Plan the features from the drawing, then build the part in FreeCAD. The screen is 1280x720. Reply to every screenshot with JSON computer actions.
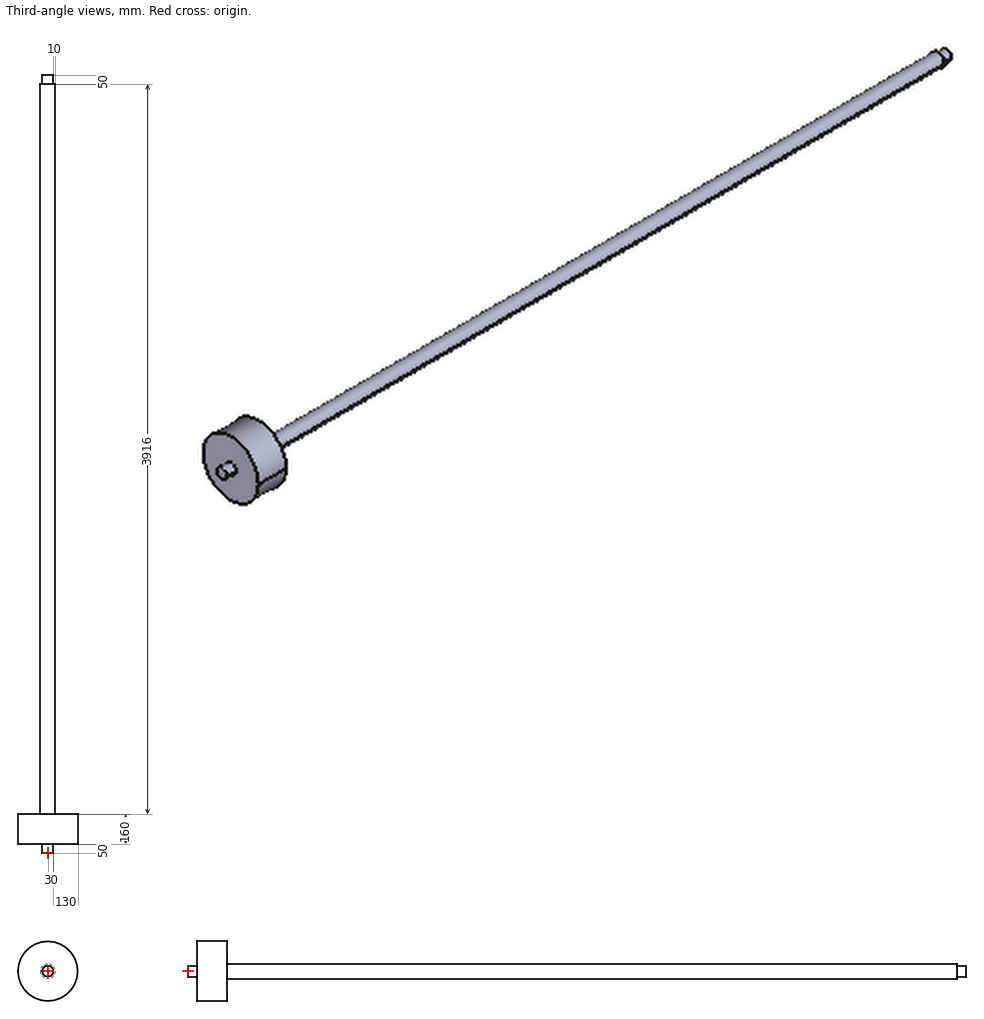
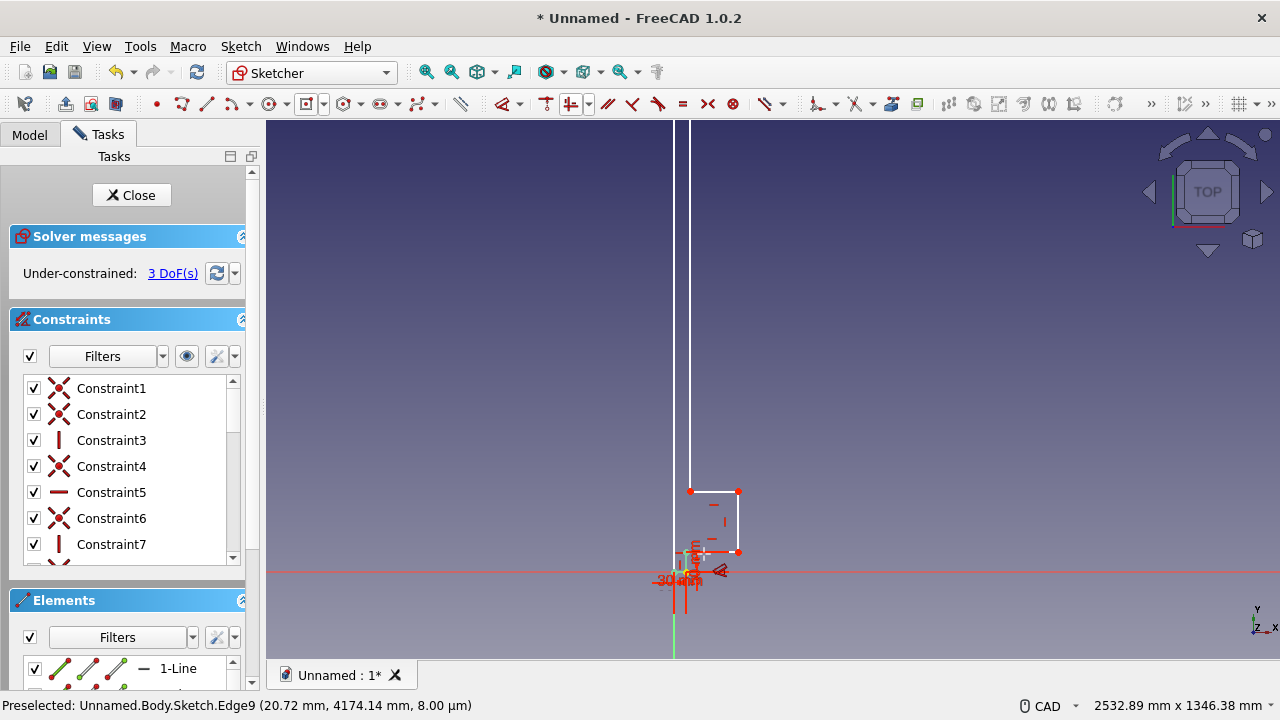
{"action": "left_click", "coordinate": [702, 552]}
{"action": "left_click", "coordinate": [712, 518]}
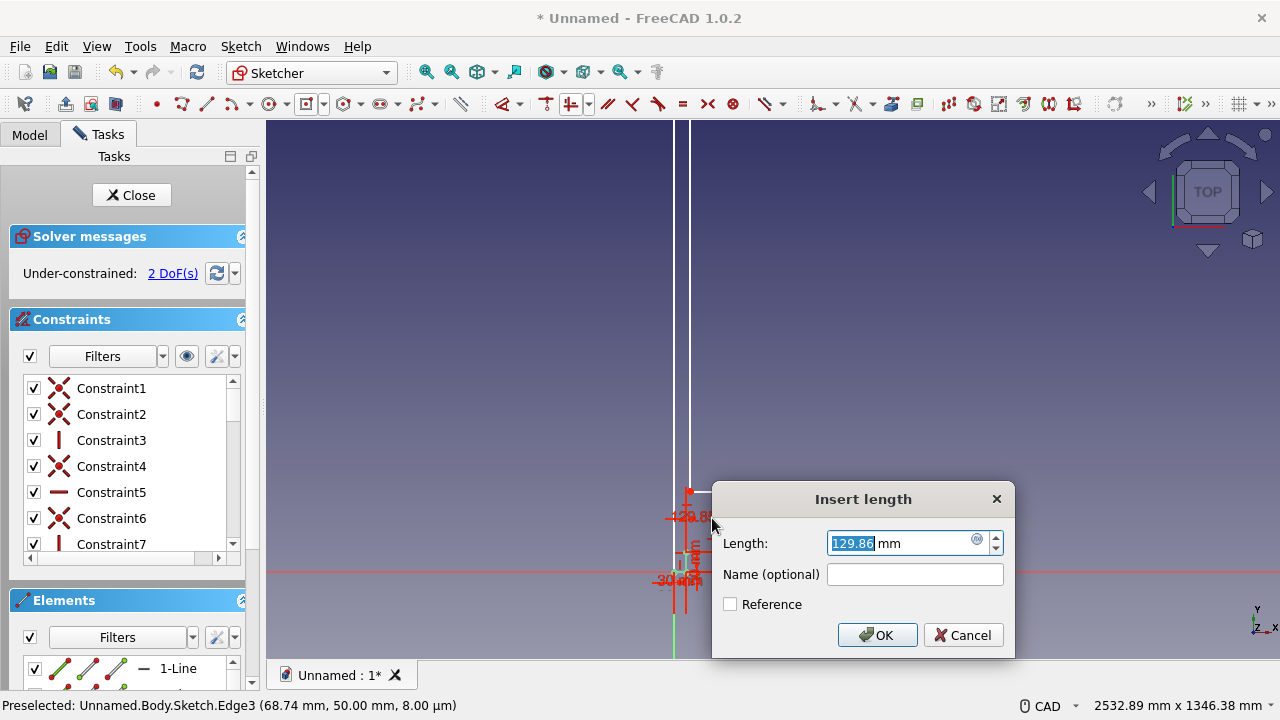
{"action": "type", "text": "130"}
{"action": "key", "text": "Return"}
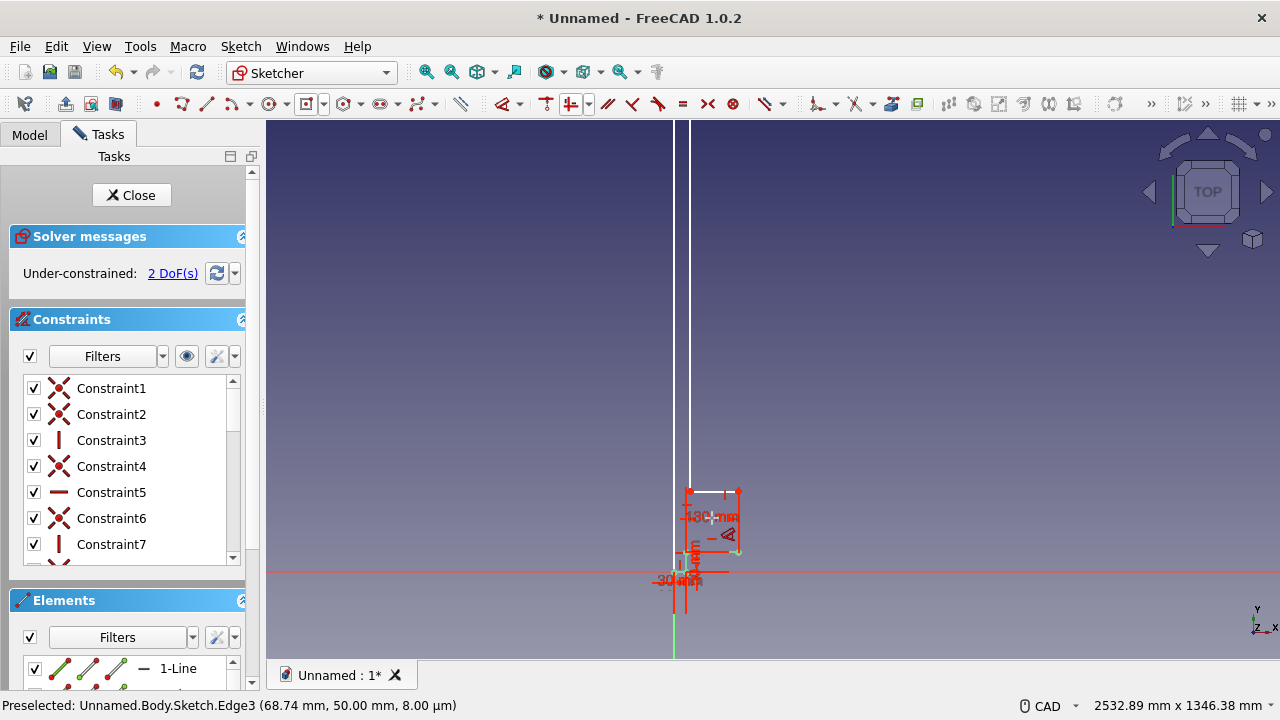
{"action": "left_click", "coordinate": [739, 534]}
{"action": "left_click", "coordinate": [773, 543]}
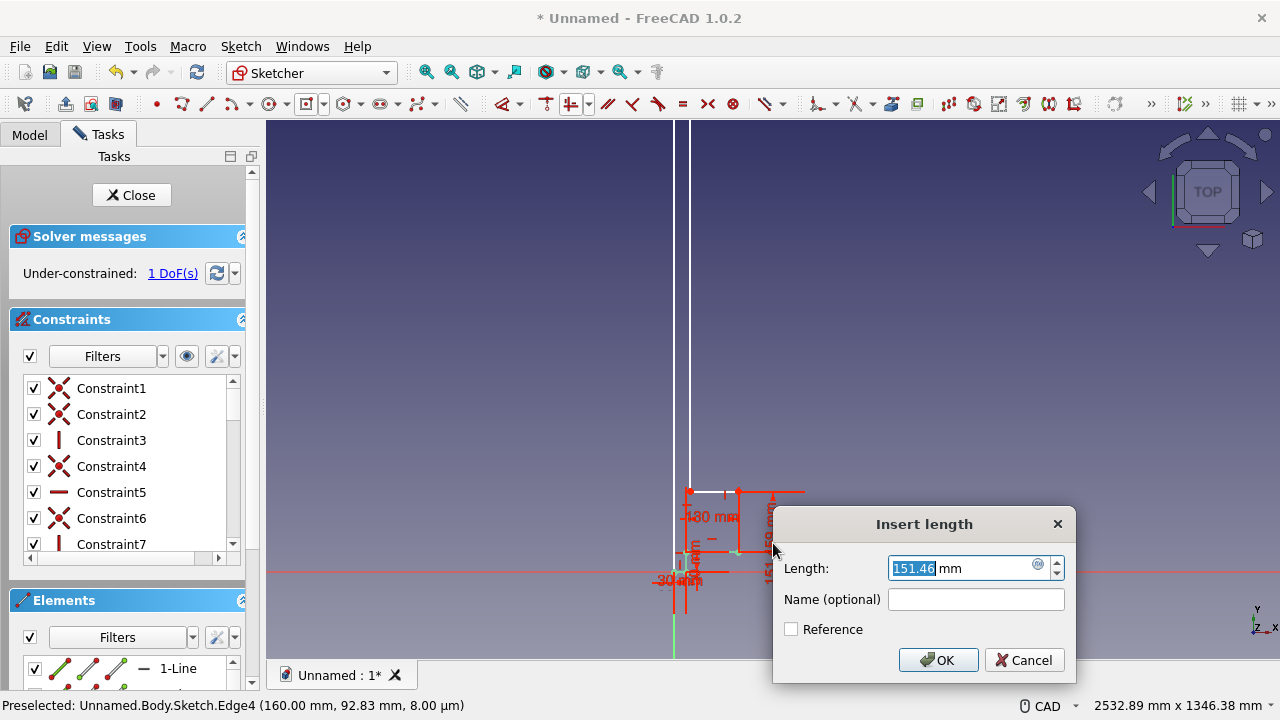
{"action": "type", "text": "160"}
{"action": "key", "text": "Return"}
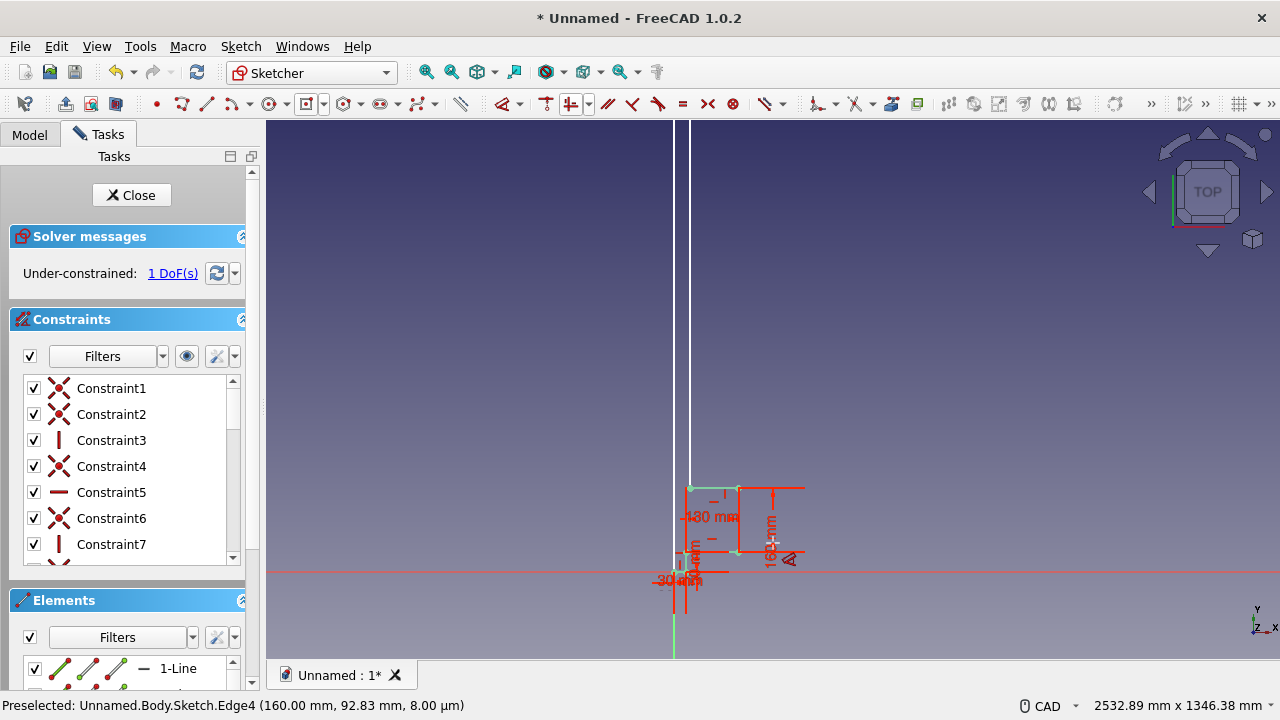
{"action": "left_click", "coordinate": [690, 175]}
{"action": "left_click", "coordinate": [656, 318]}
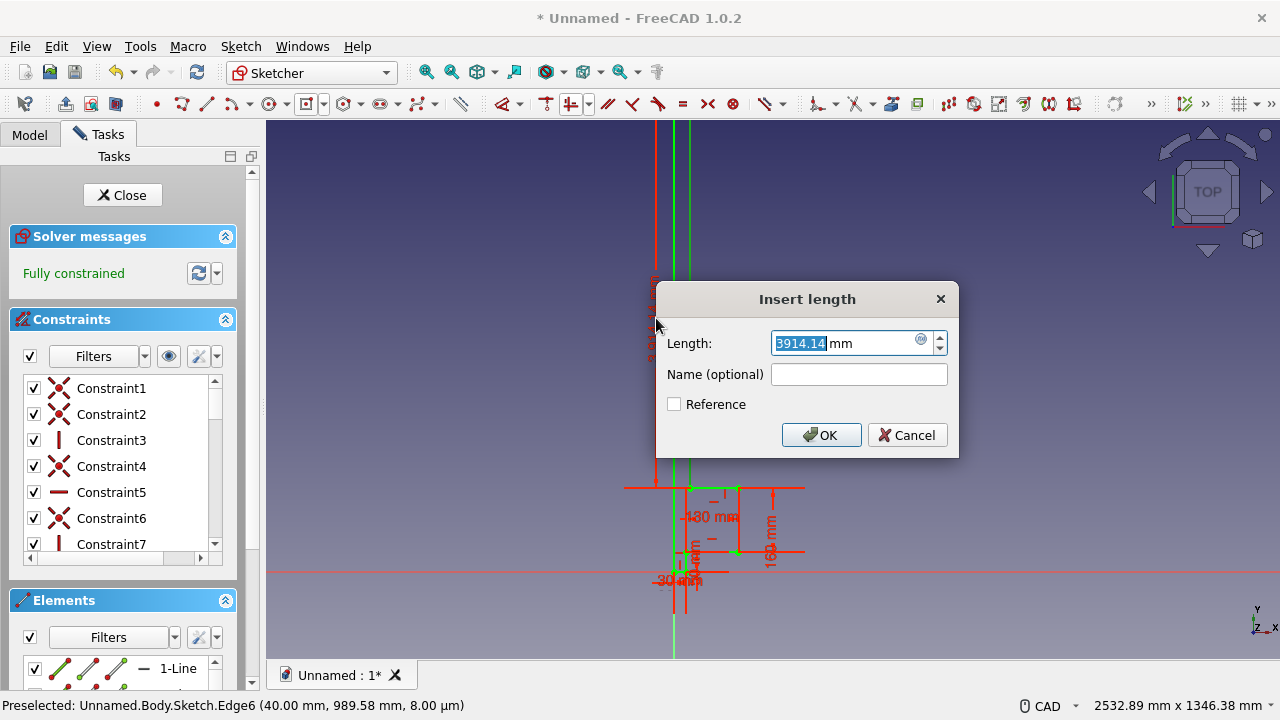
{"action": "type", "text": "3916"}
{"action": "key", "text": "Return"}
{"action": "key", "text": "Escape"}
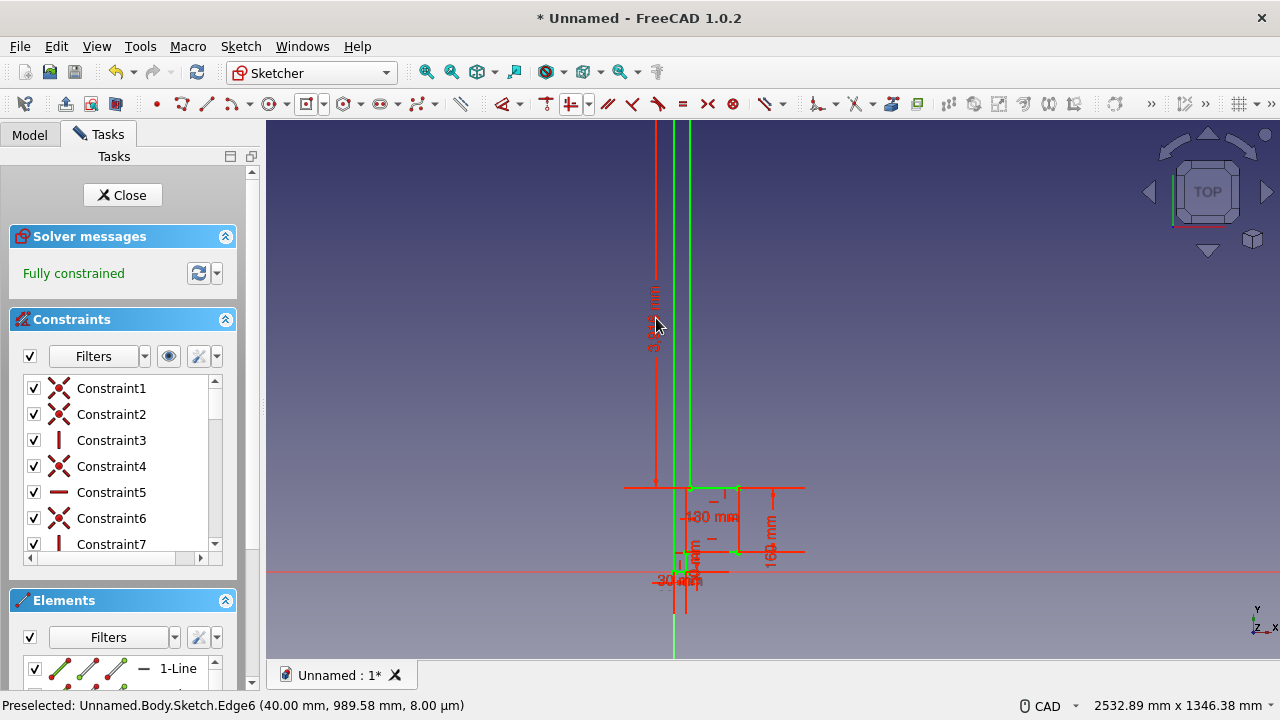
{"action": "left_click", "coordinate": [123, 195]}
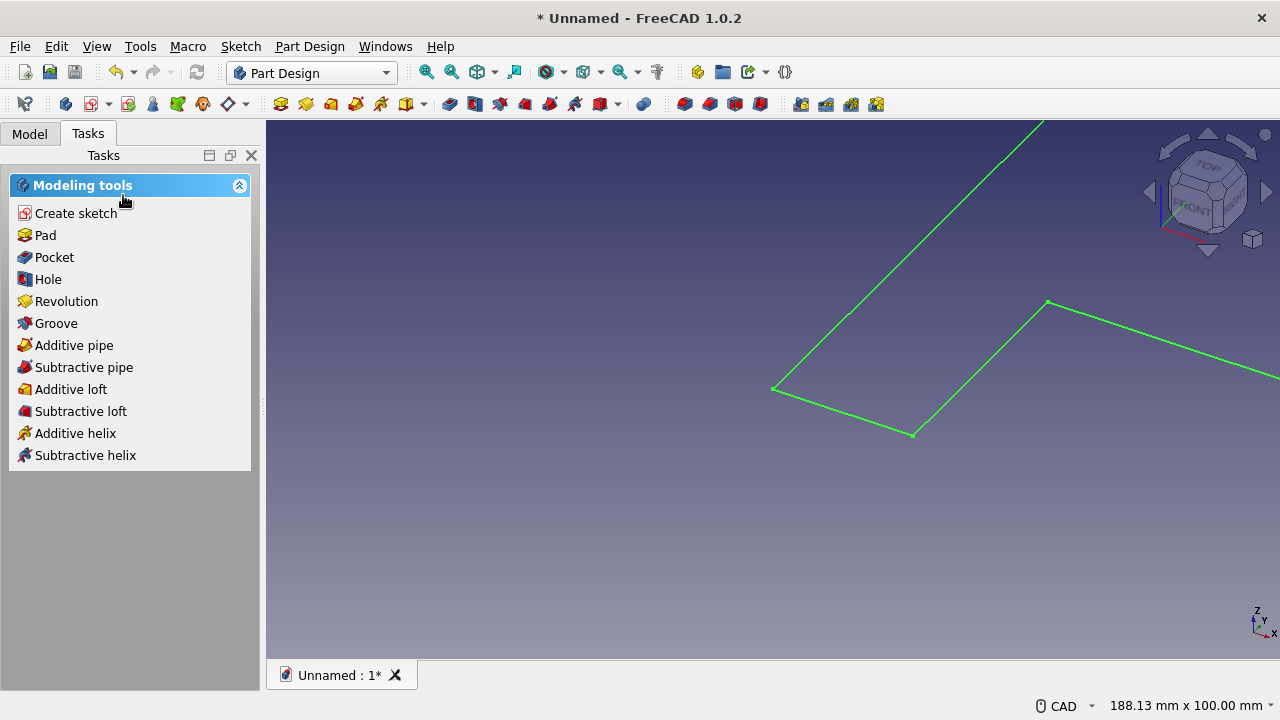
{"action": "left_click", "coordinate": [306, 104]}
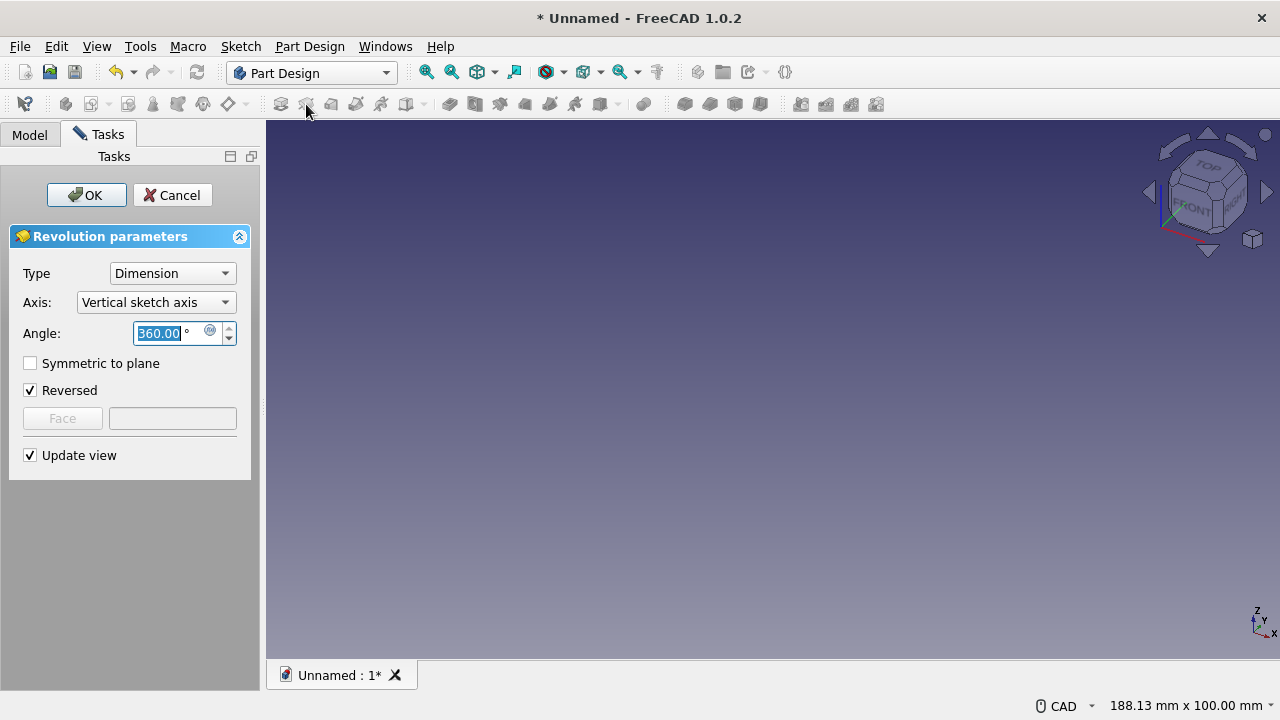
{"action": "left_click", "coordinate": [87, 195]}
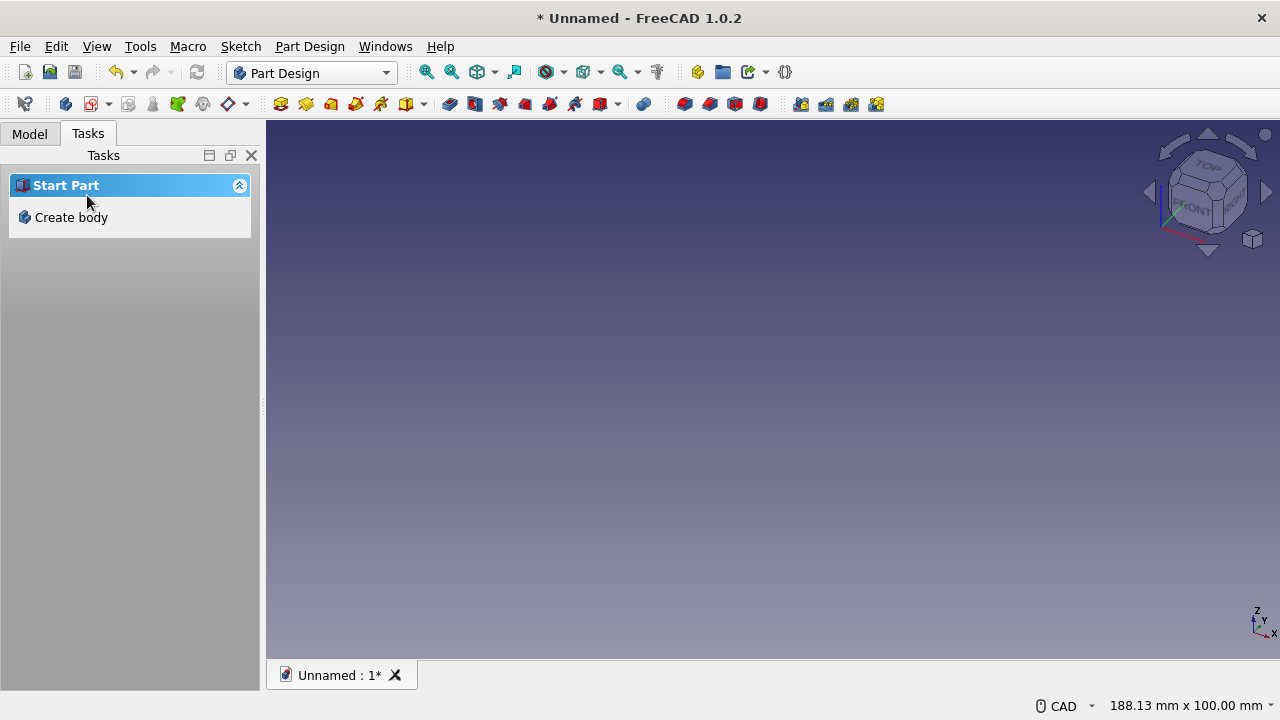
{"action": "key", "text": "0"}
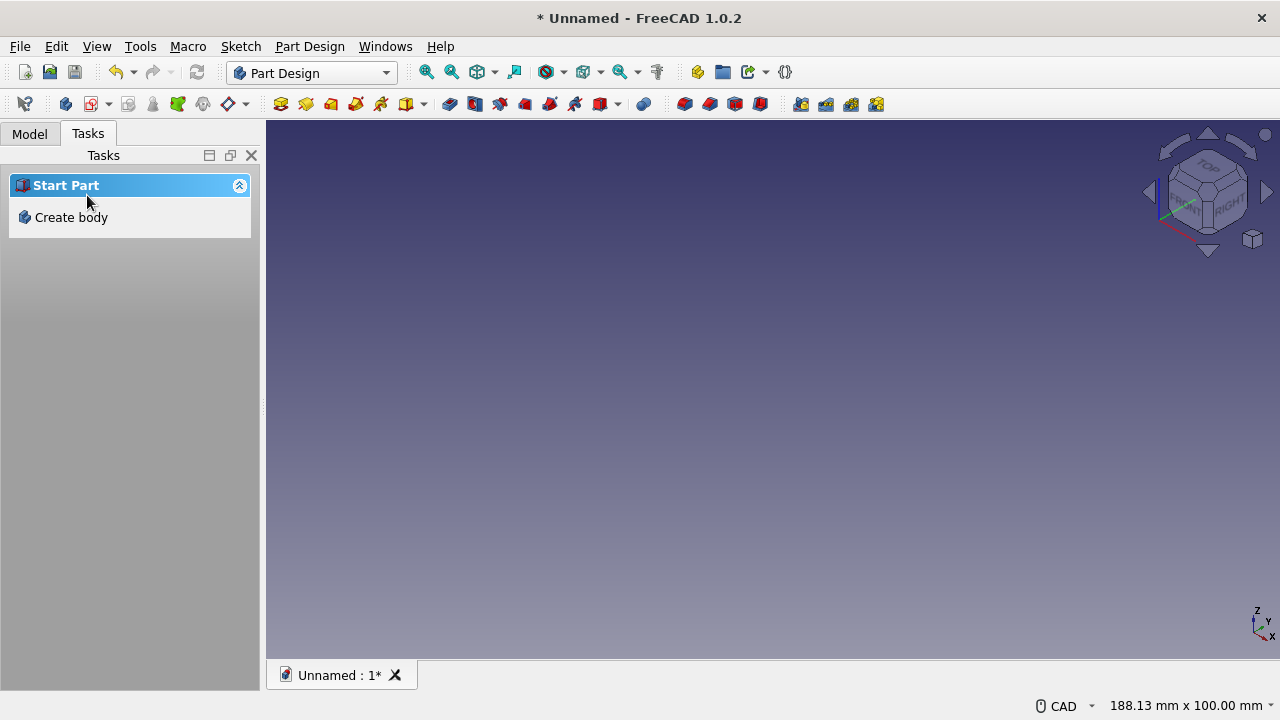
{"action": "left_click", "coordinate": [427, 72]}